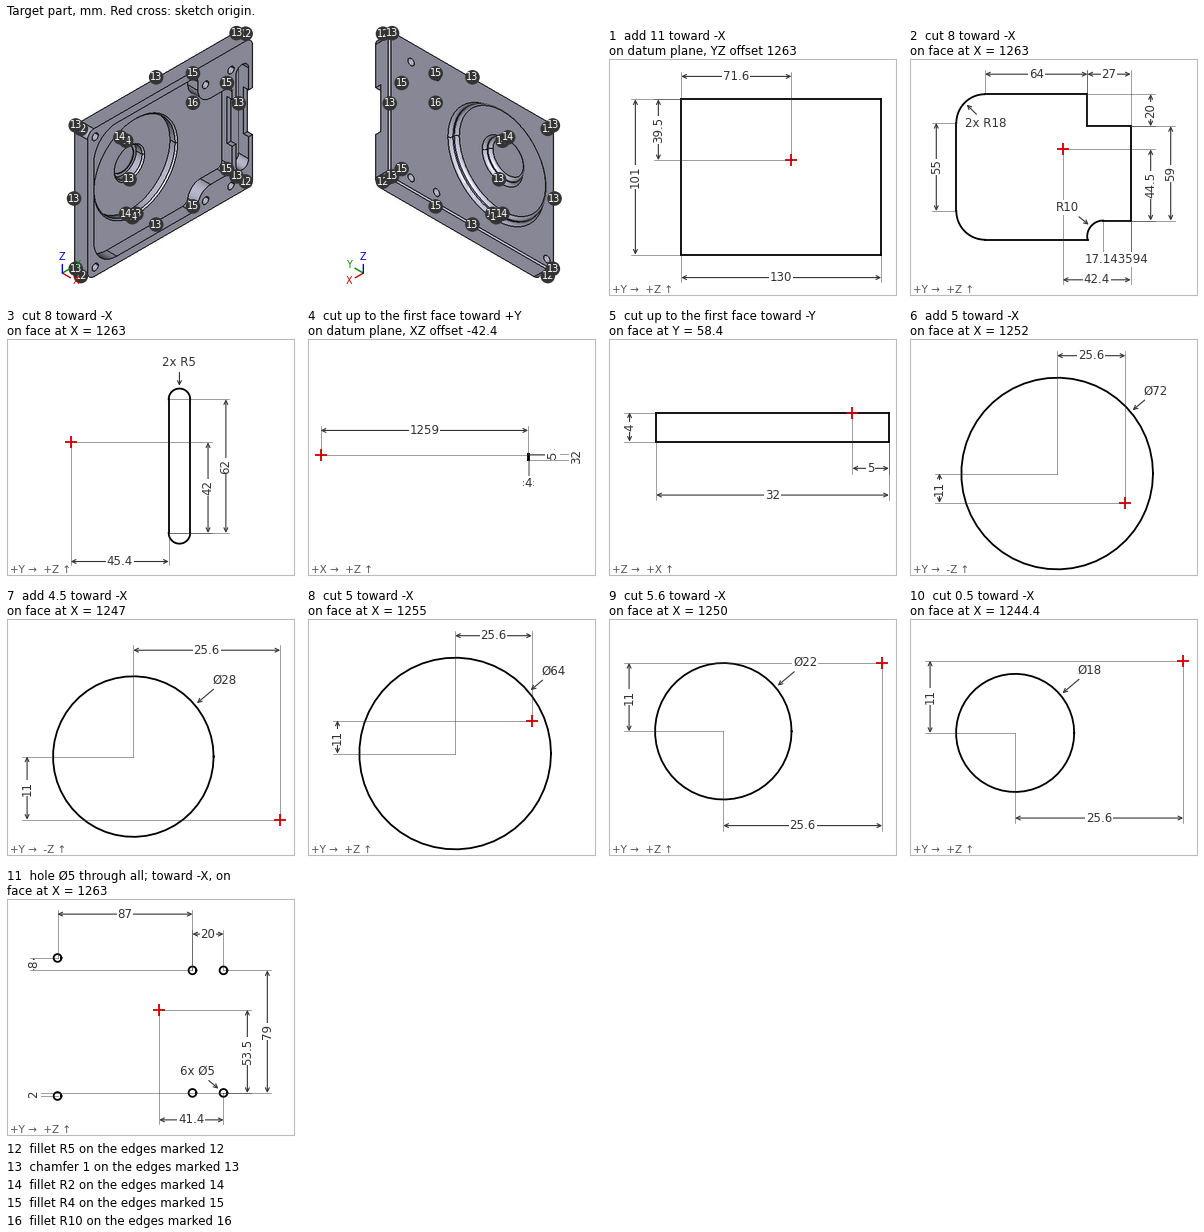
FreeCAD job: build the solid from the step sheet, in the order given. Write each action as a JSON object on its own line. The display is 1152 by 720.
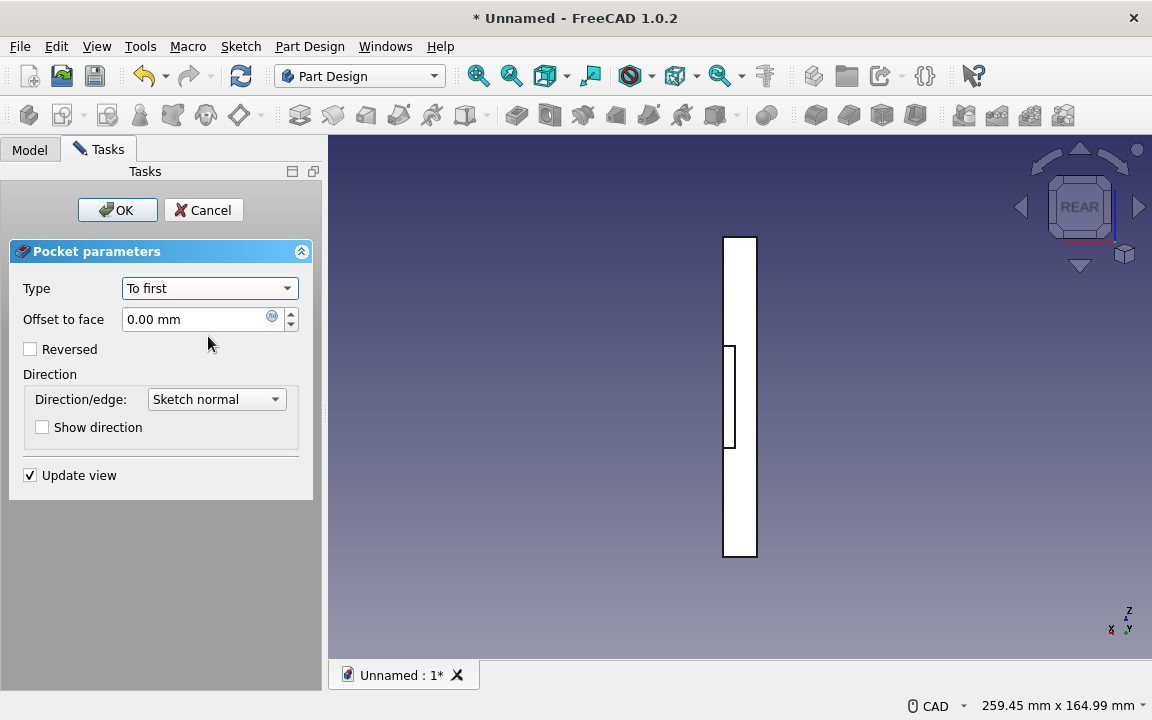
{"action": "left_click", "coordinate": [118, 210]}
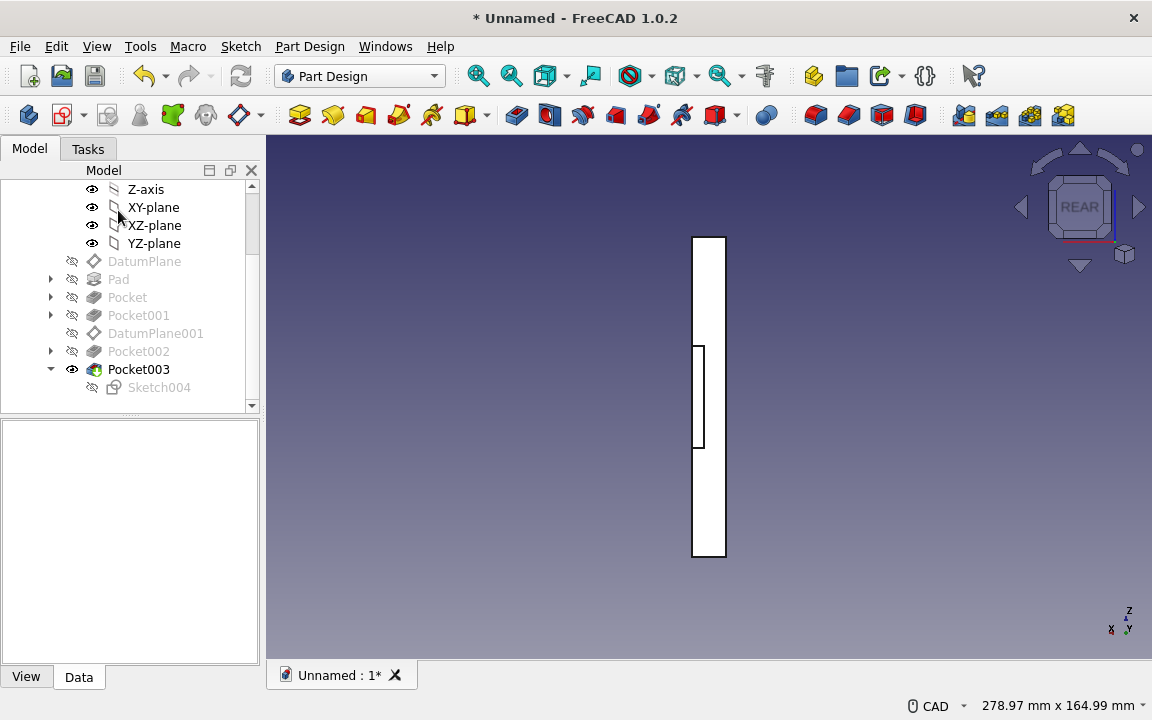
{"action": "key", "text": "6"}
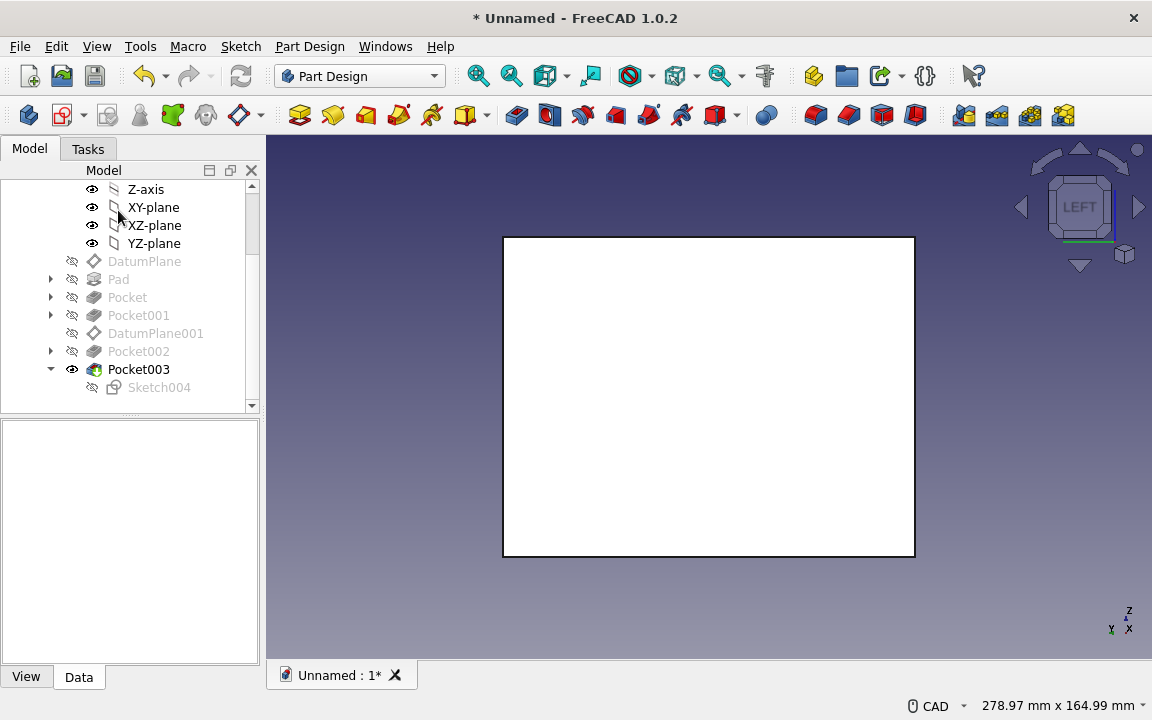
{"action": "left_click", "coordinate": [709, 396]}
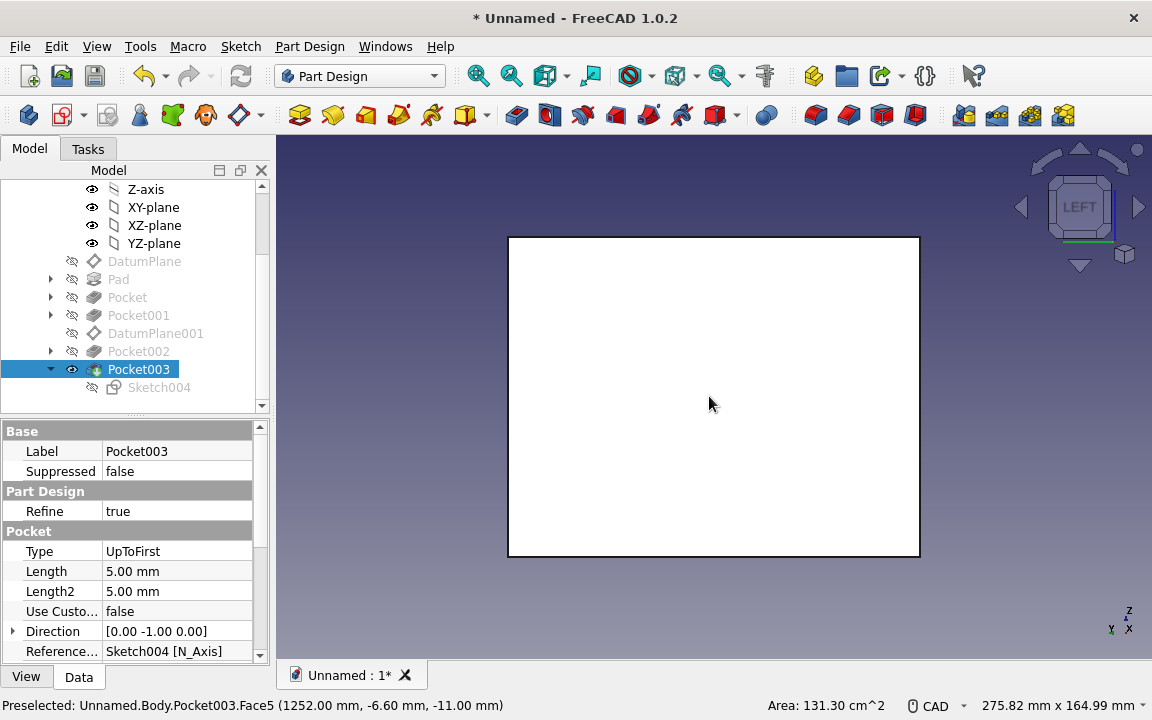
{"action": "left_click", "coordinate": [62, 116]}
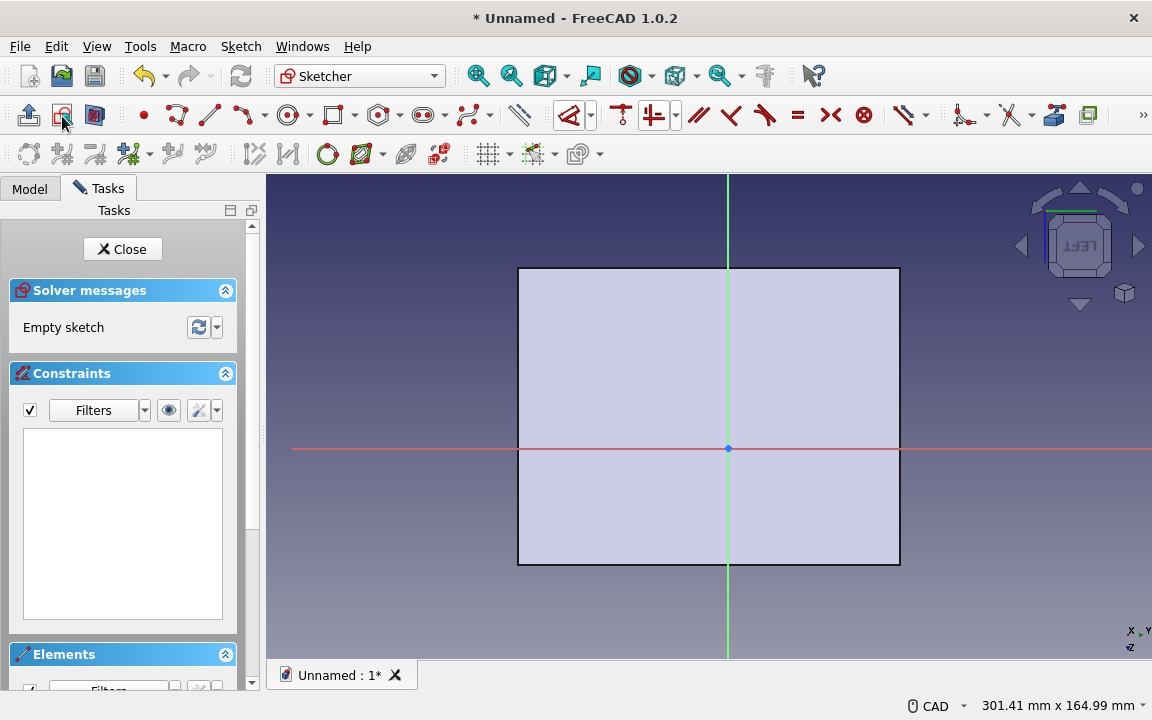
{"action": "scroll", "coordinate": [679, 416], "scroll_direction": "up", "scroll_amount": 2}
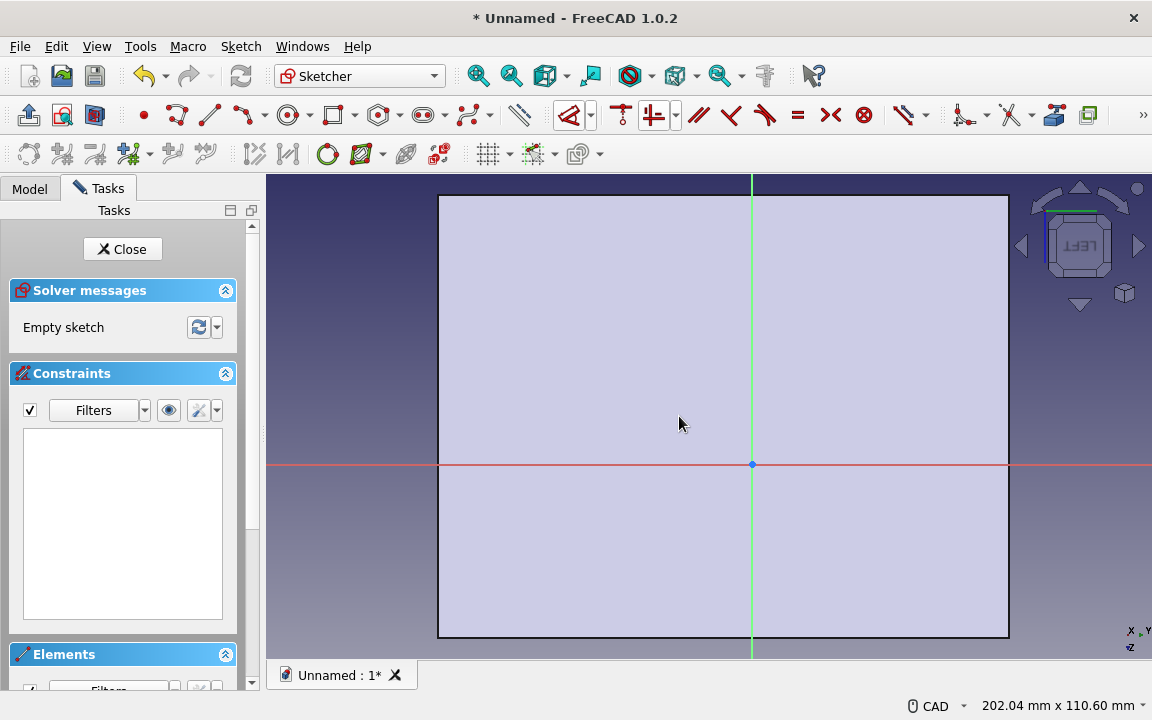
{"action": "left_click", "coordinate": [288, 116]}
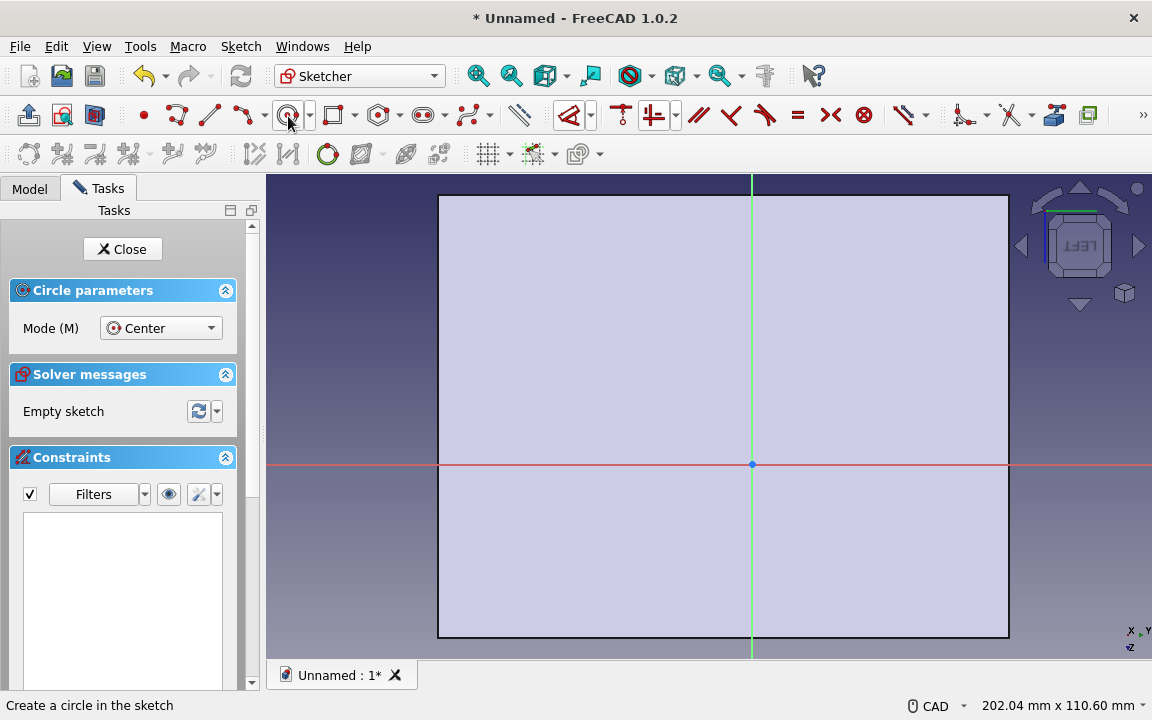
{"action": "left_click", "coordinate": [640, 416]}
{"action": "left_click", "coordinate": [529, 305]}
{"action": "key", "text": "Escape"}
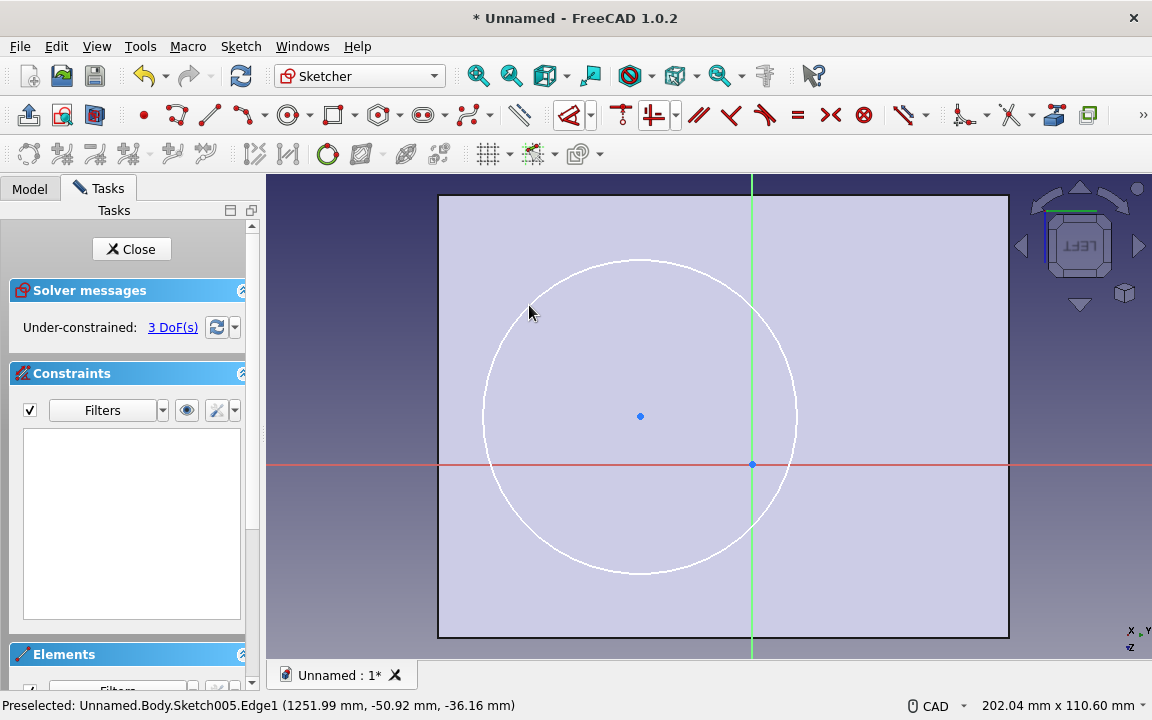
{"action": "left_click", "coordinate": [751, 306]}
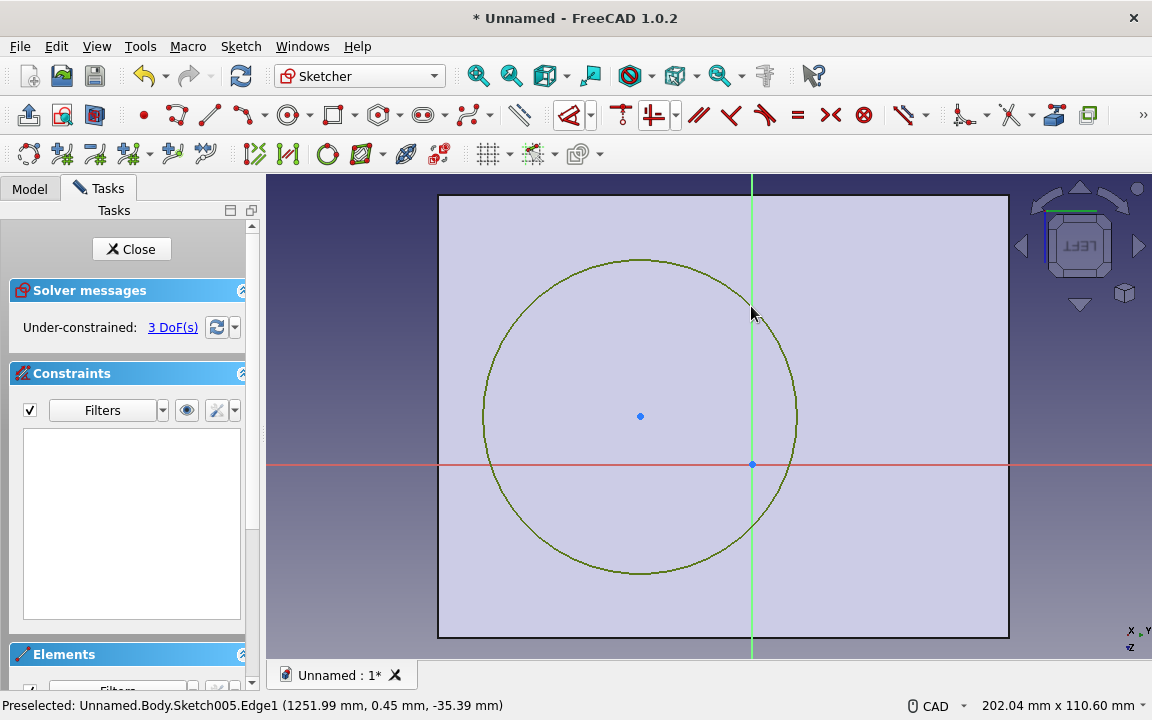
{"action": "key", "text": "k o"}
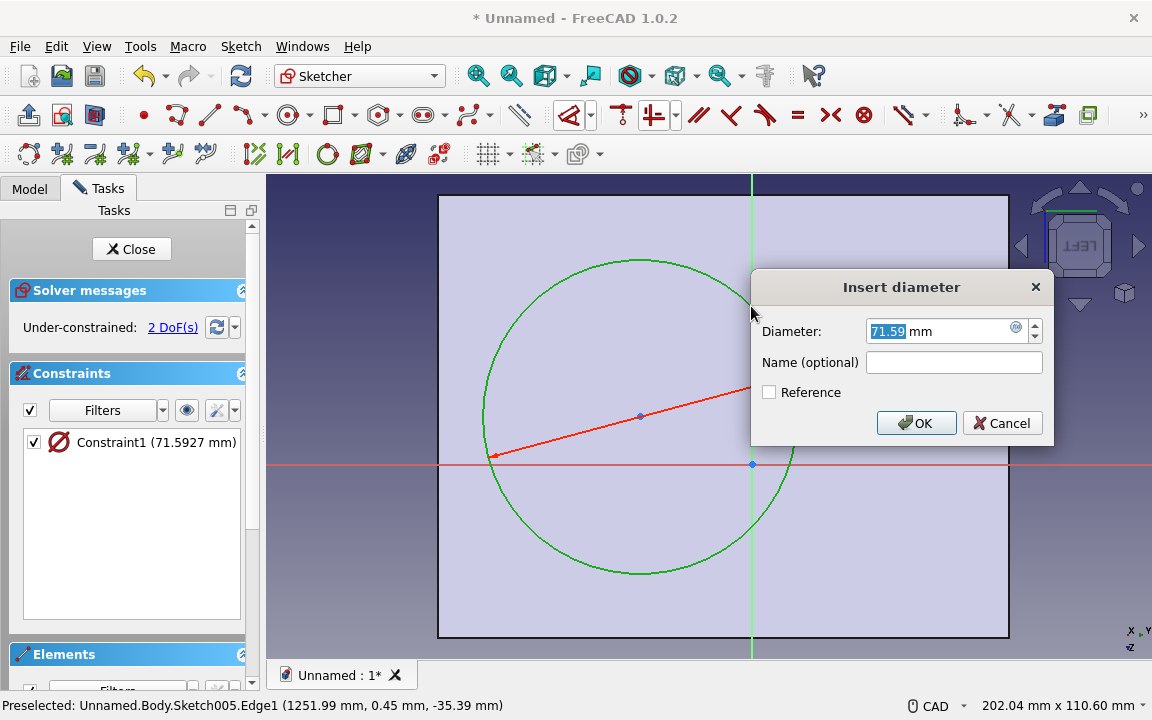
{"action": "type", "text": "72"}
{"action": "key", "text": "Return"}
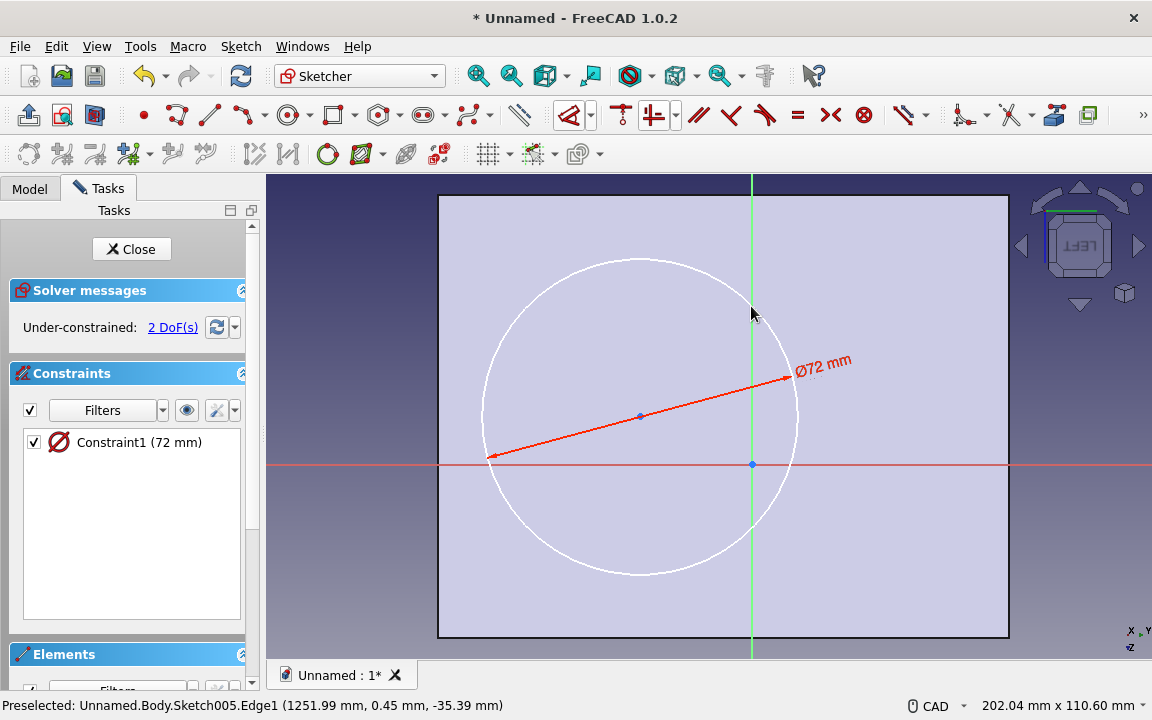
{"action": "left_click", "coordinate": [640, 417]}